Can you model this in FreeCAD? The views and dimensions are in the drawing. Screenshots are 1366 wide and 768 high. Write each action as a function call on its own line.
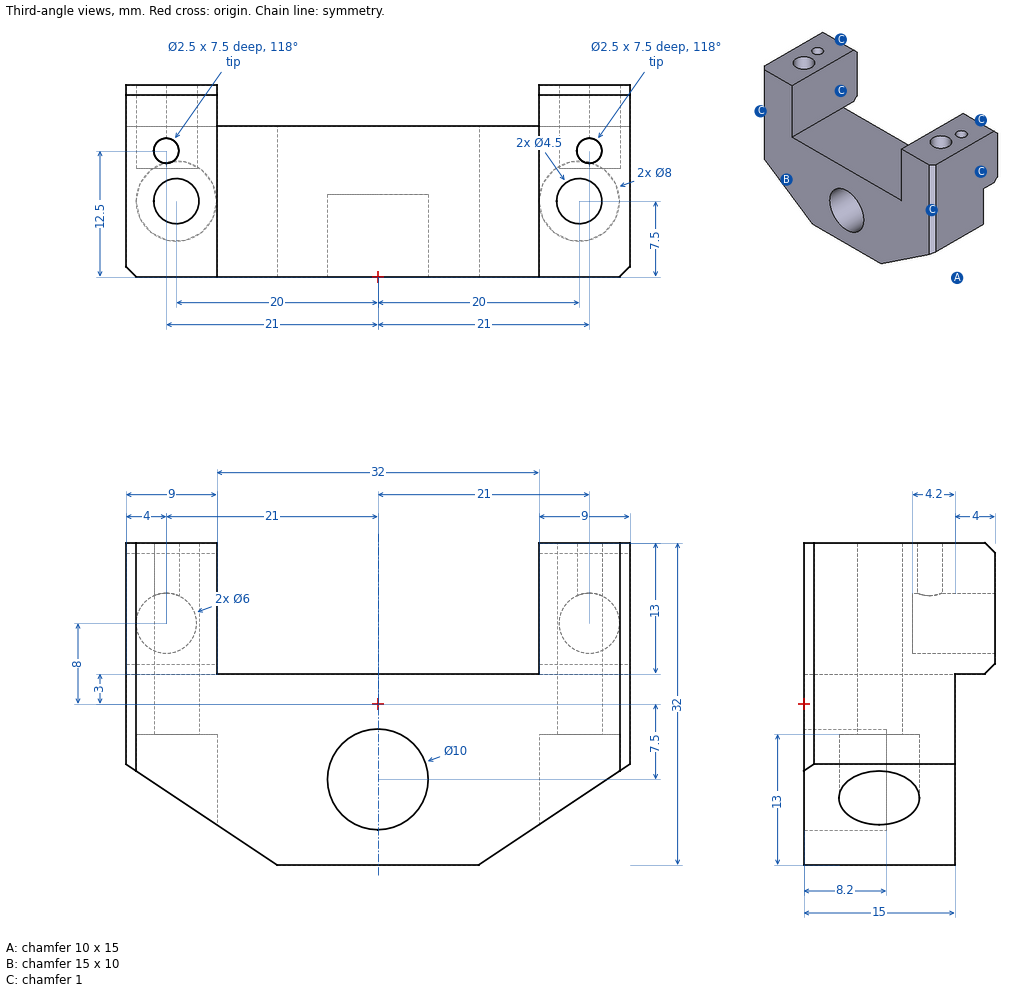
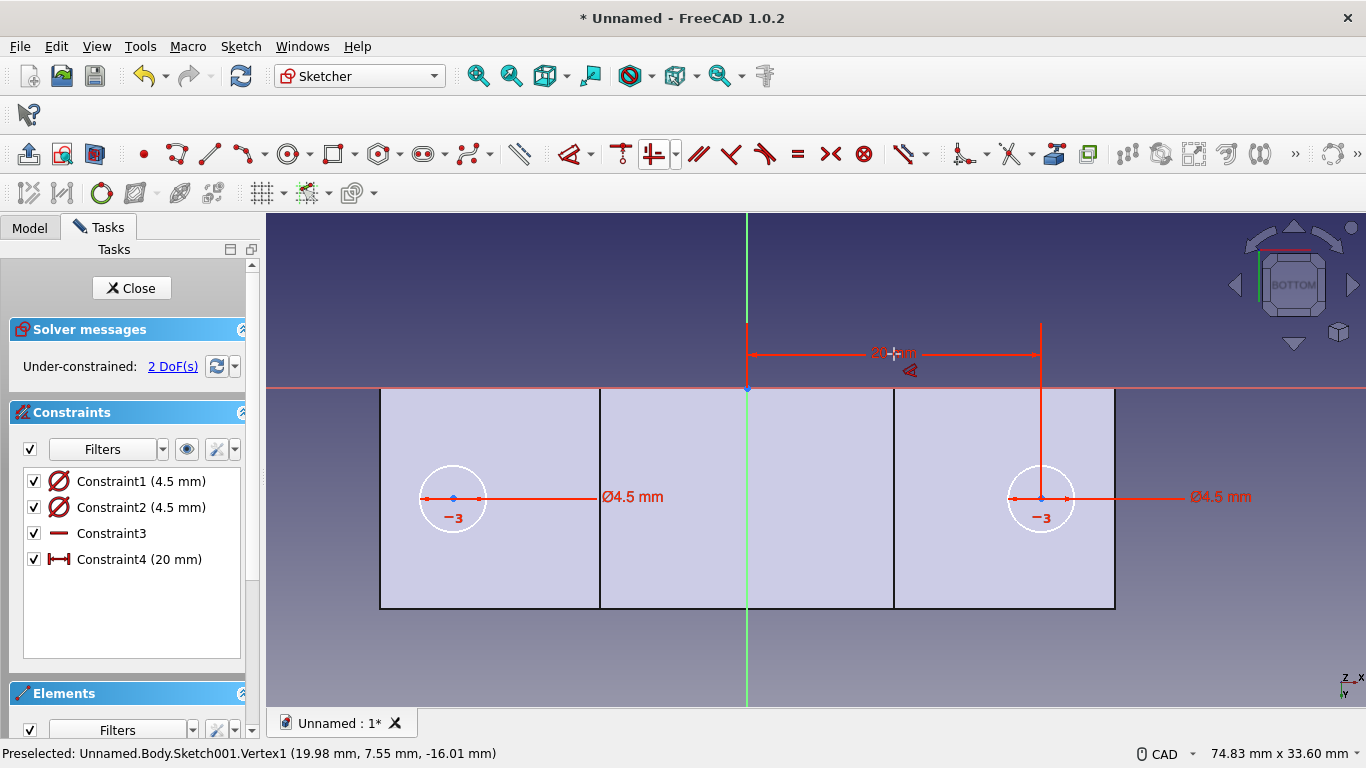
click(453, 499)
click(600, 354)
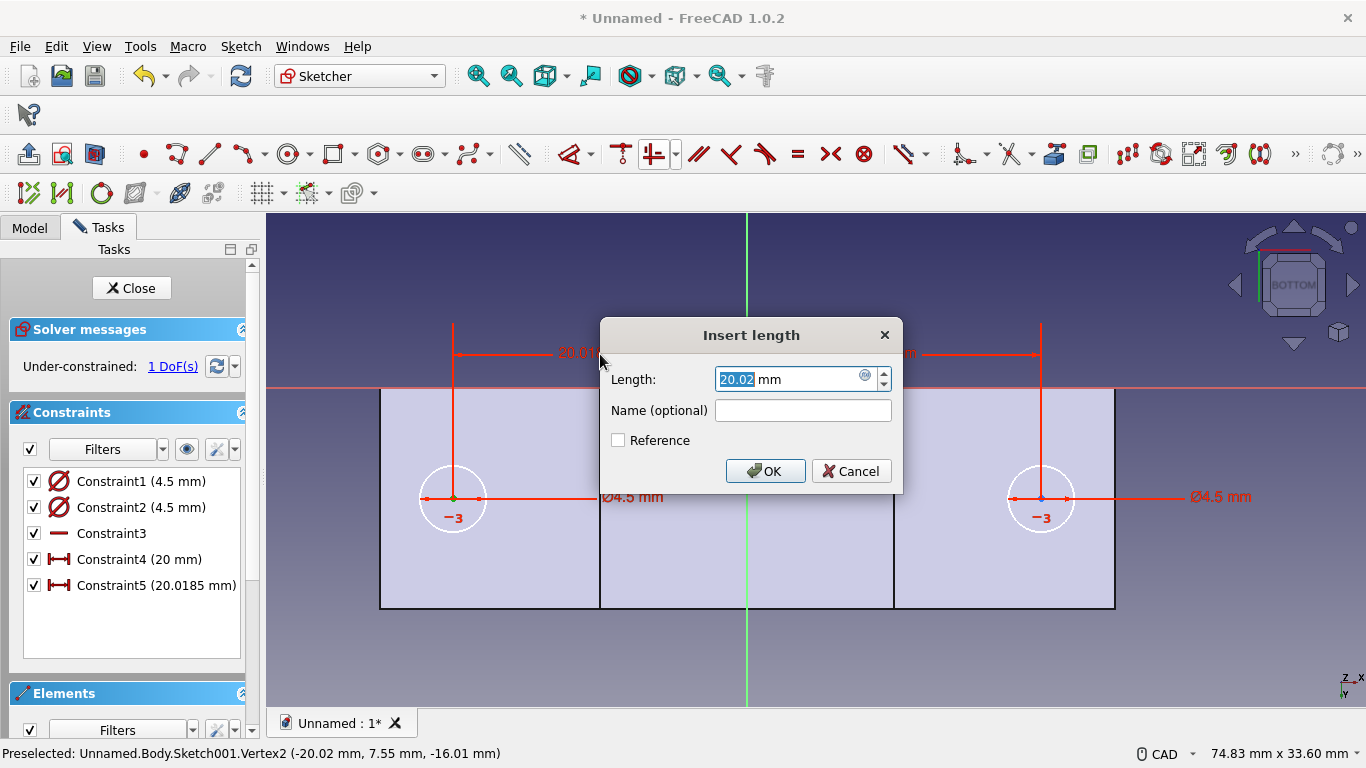
text(20)
key(Return)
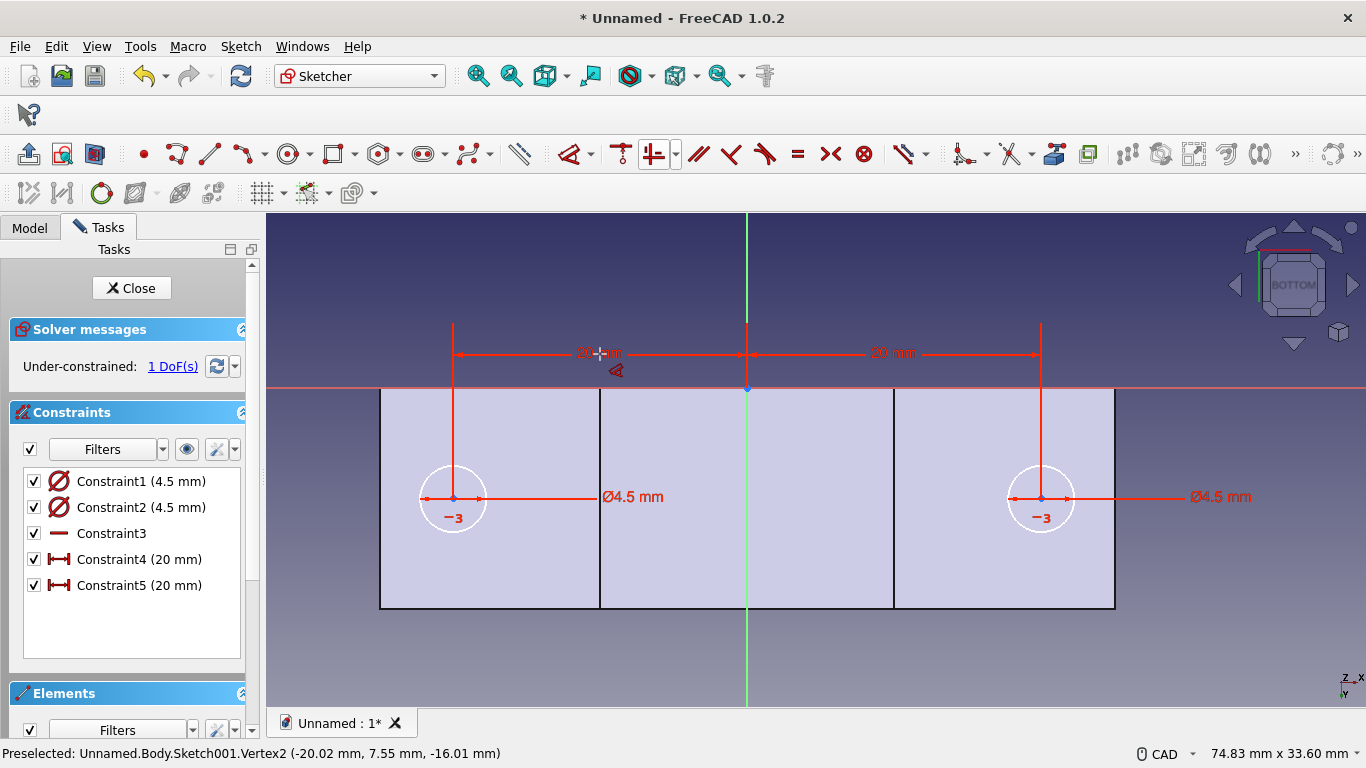
click(1041, 499)
click(1075, 444)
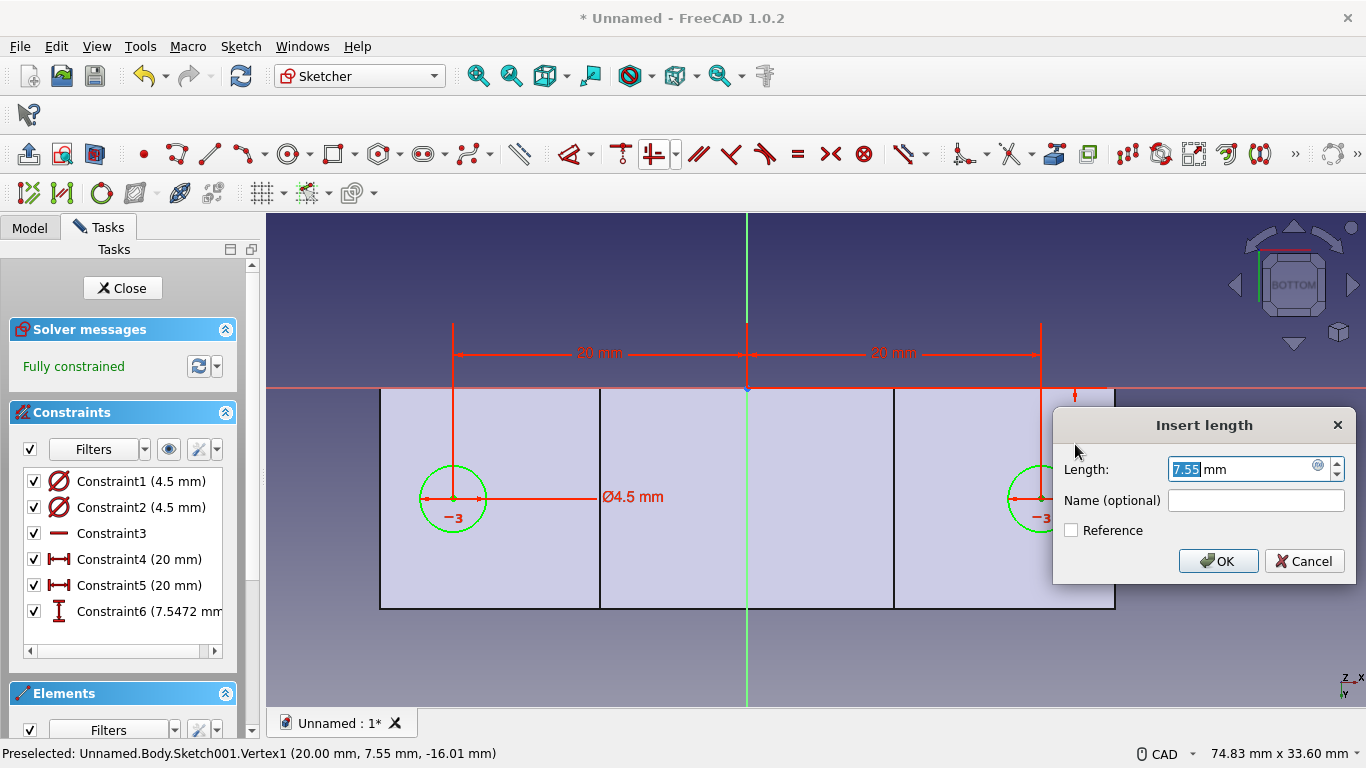
text(7.5)
key(Return)
key(Escape)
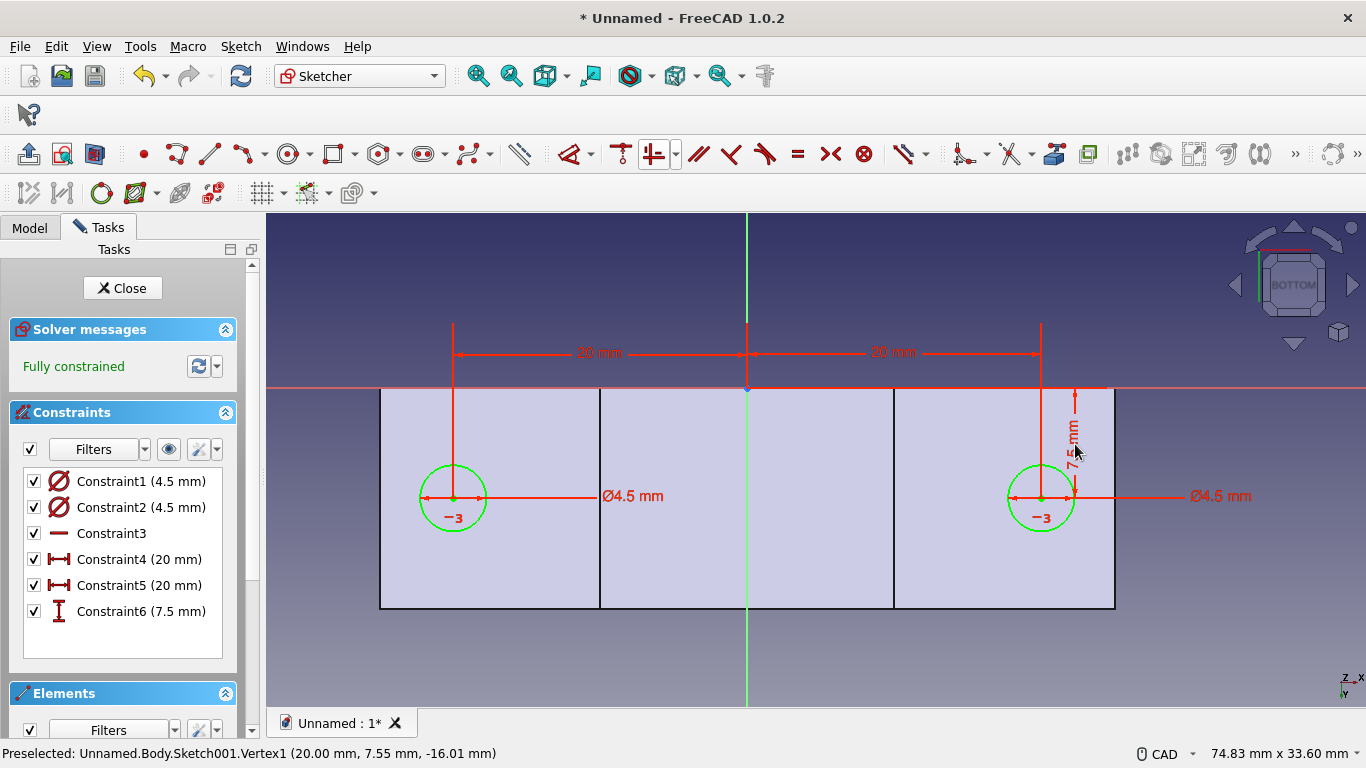
click(123, 288)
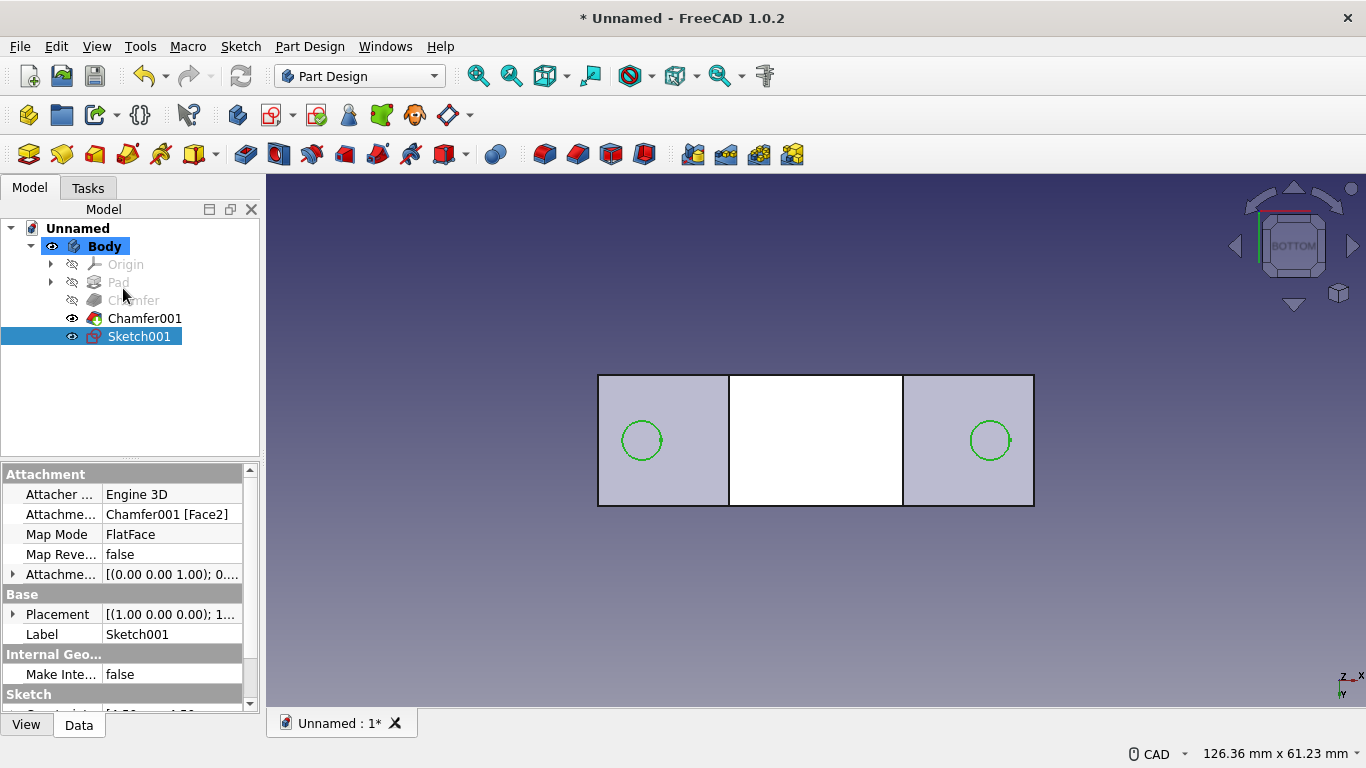
click(246, 154)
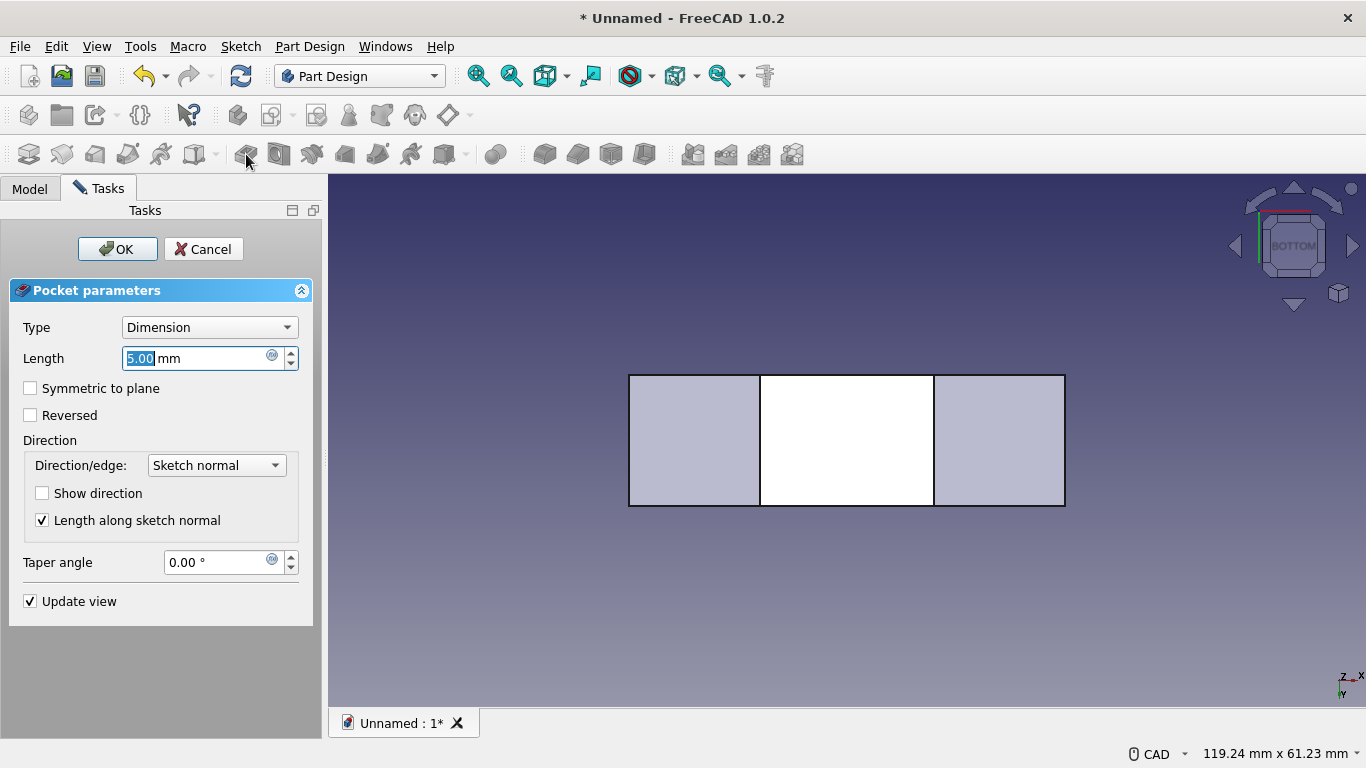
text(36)
key(Tab)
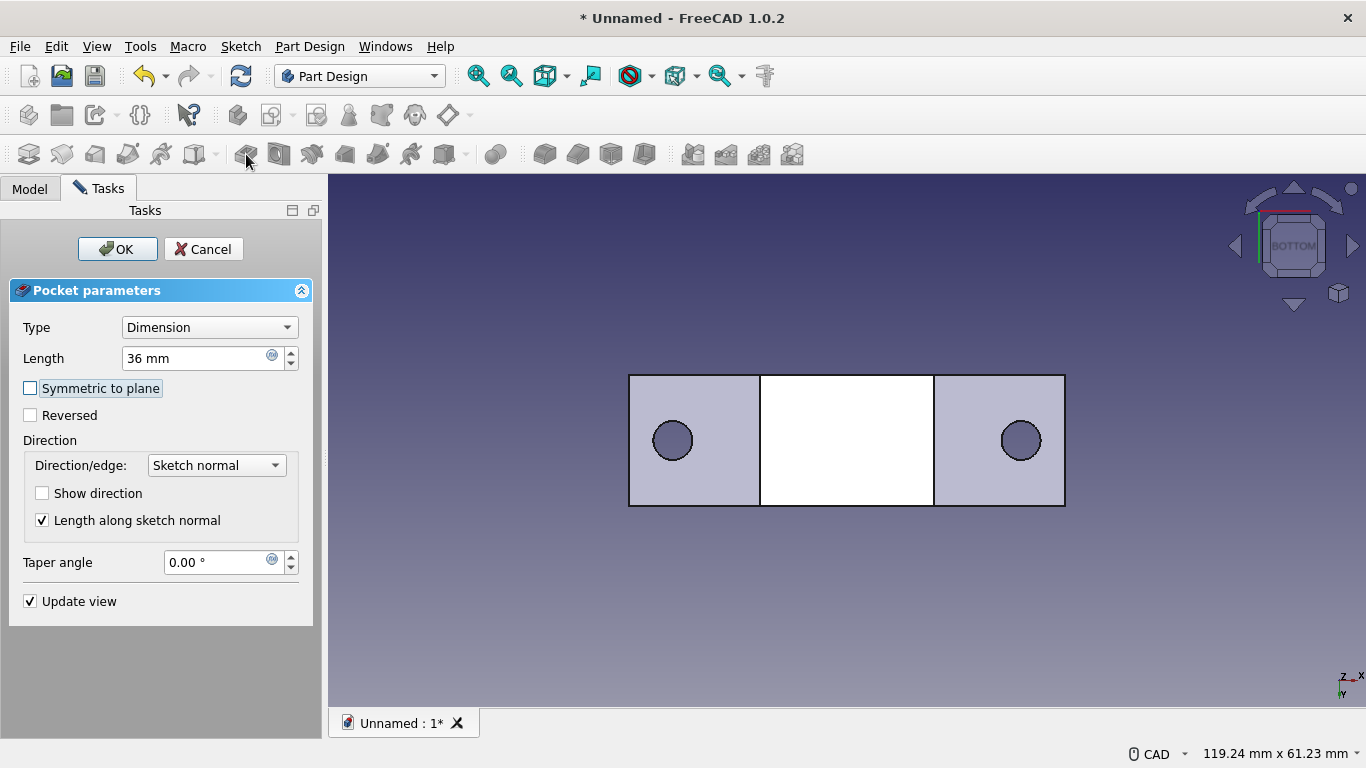
click(118, 249)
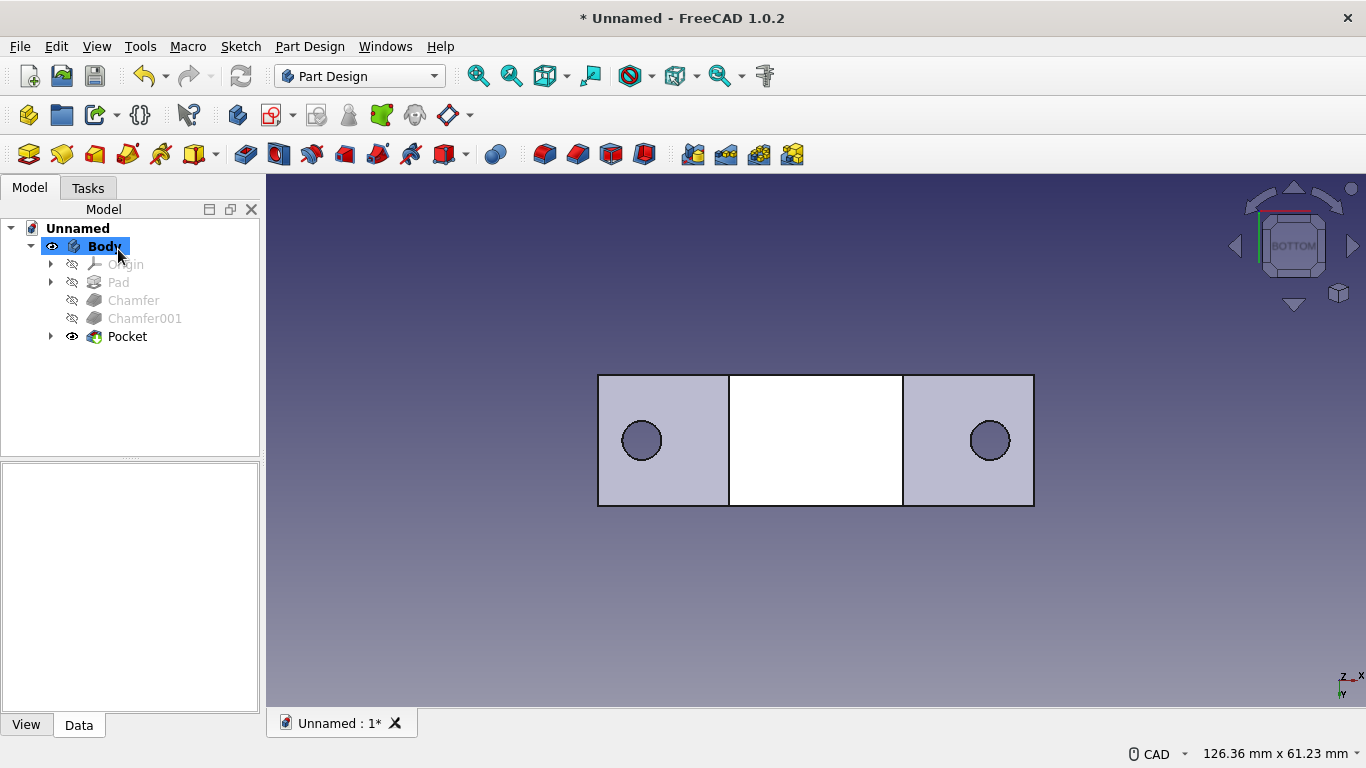
click(479, 76)